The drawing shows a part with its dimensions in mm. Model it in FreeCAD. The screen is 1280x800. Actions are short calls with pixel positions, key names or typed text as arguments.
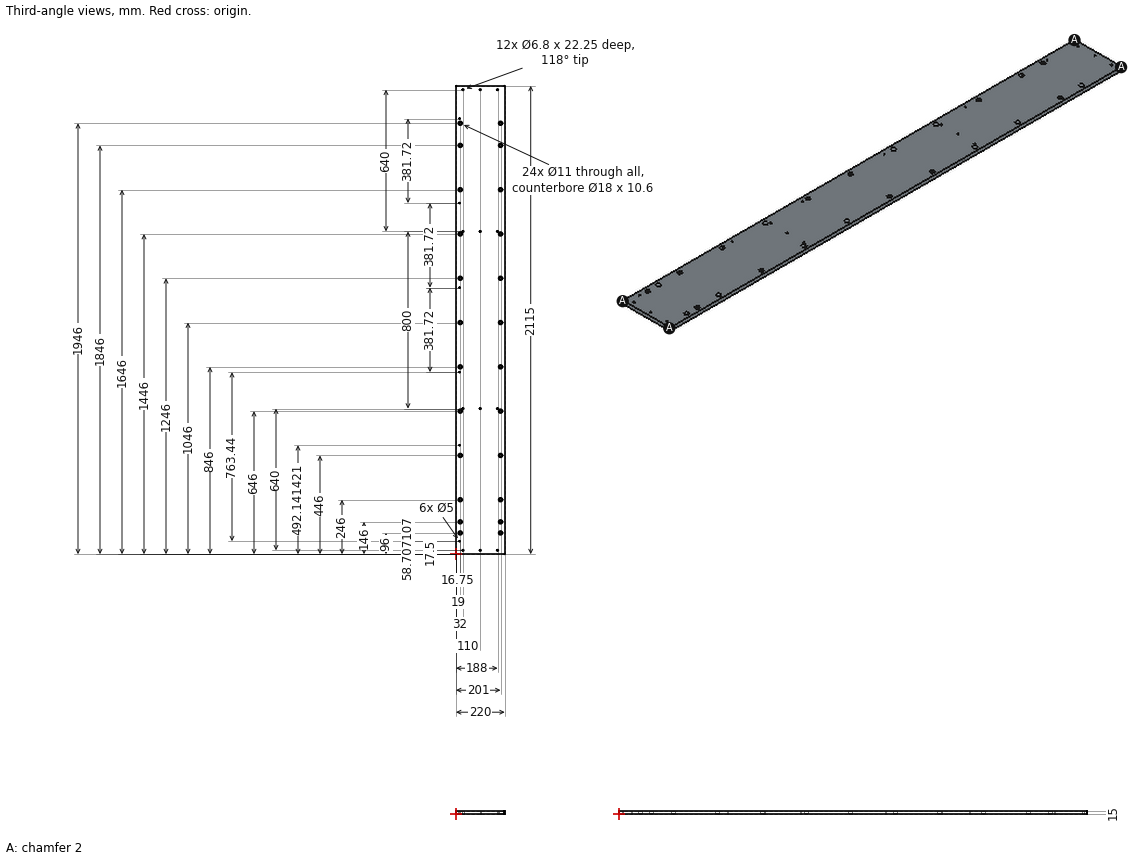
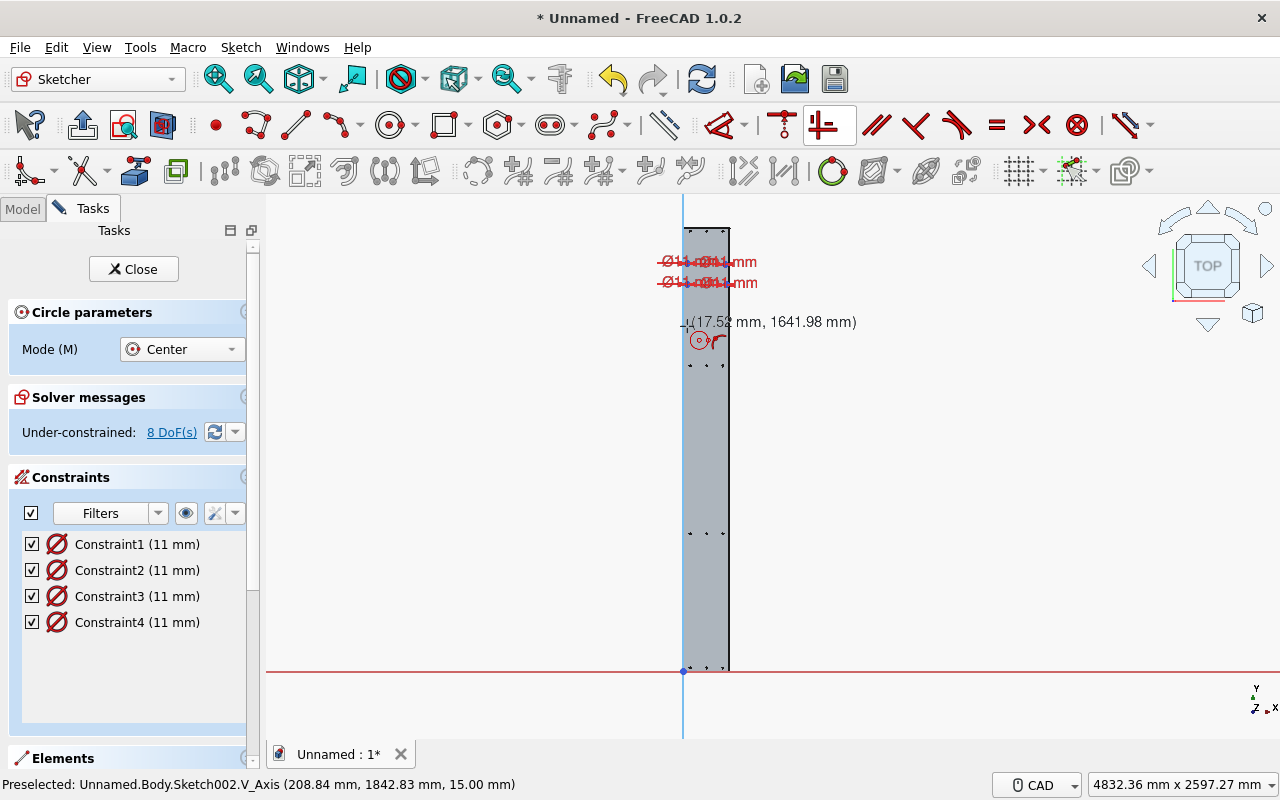
scroll(687, 326, up, 7)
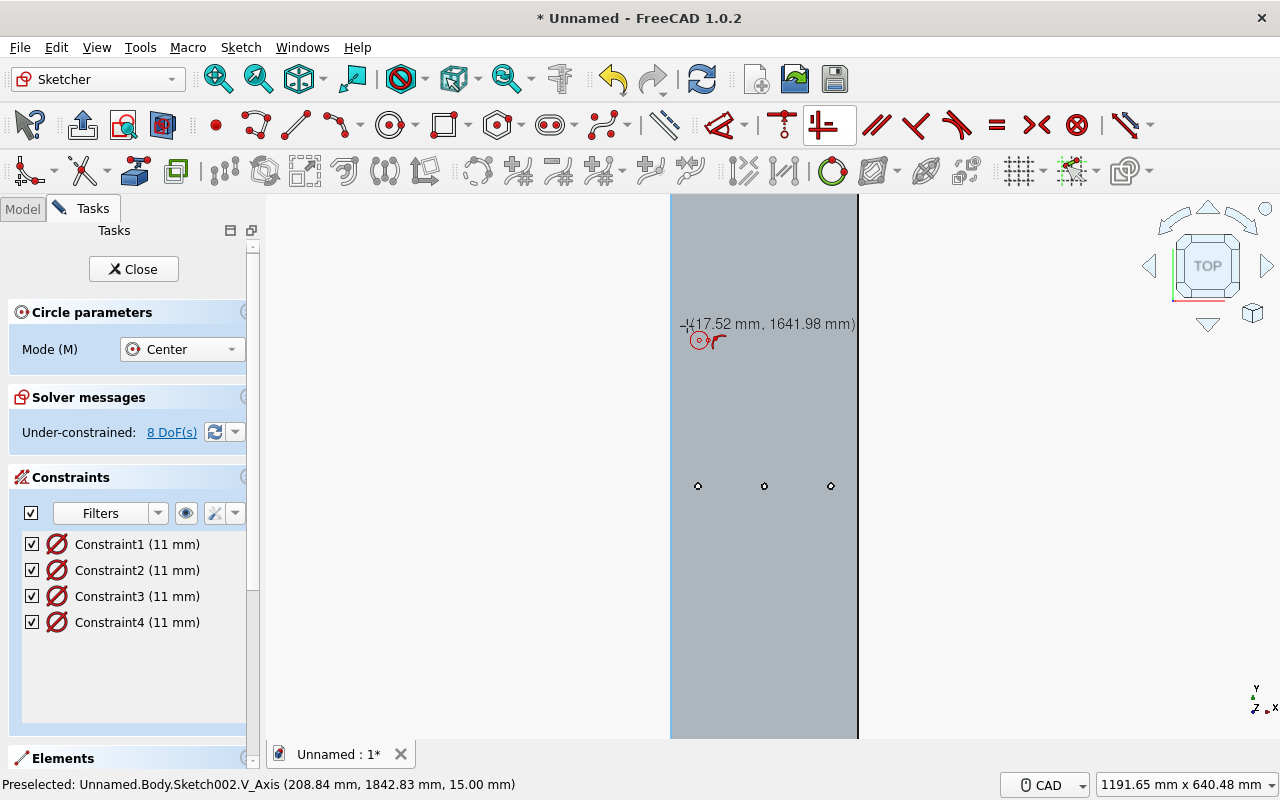
click(687, 326)
move(690, 323)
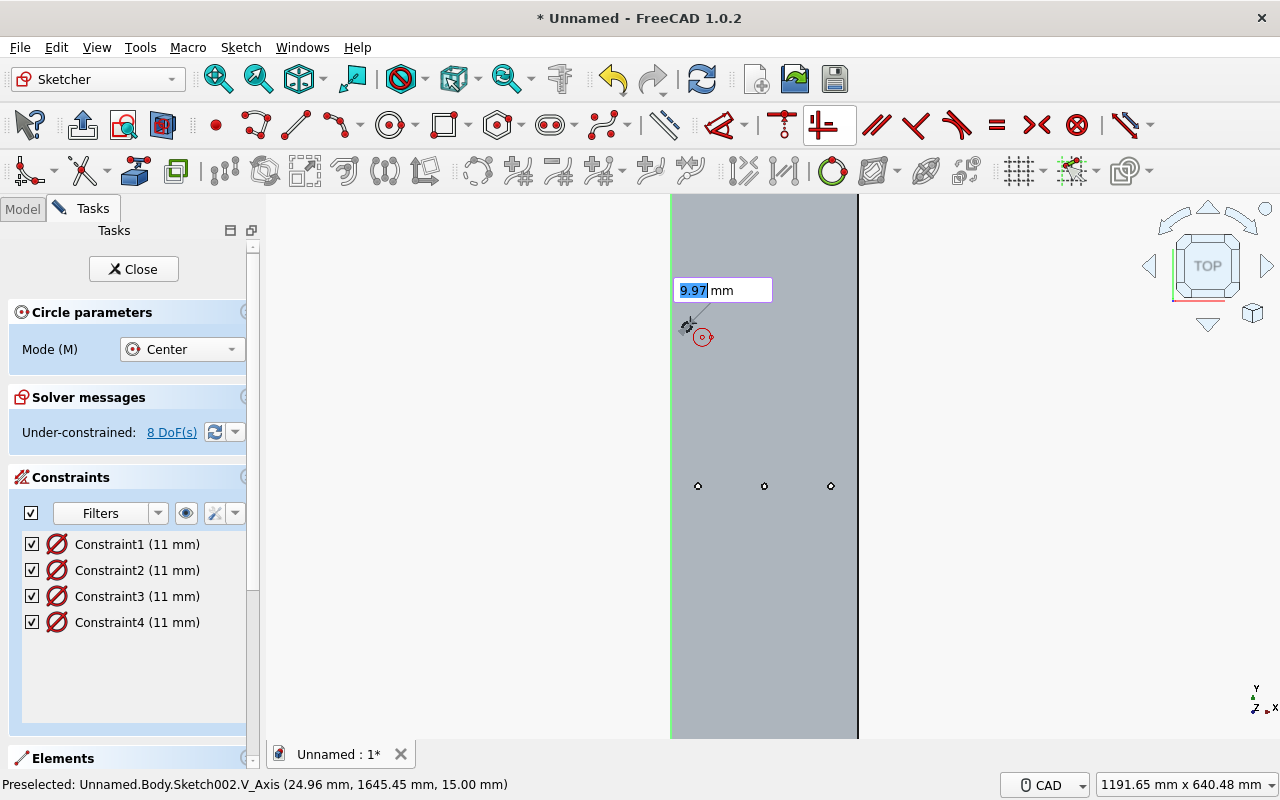
text(11)
key(Return)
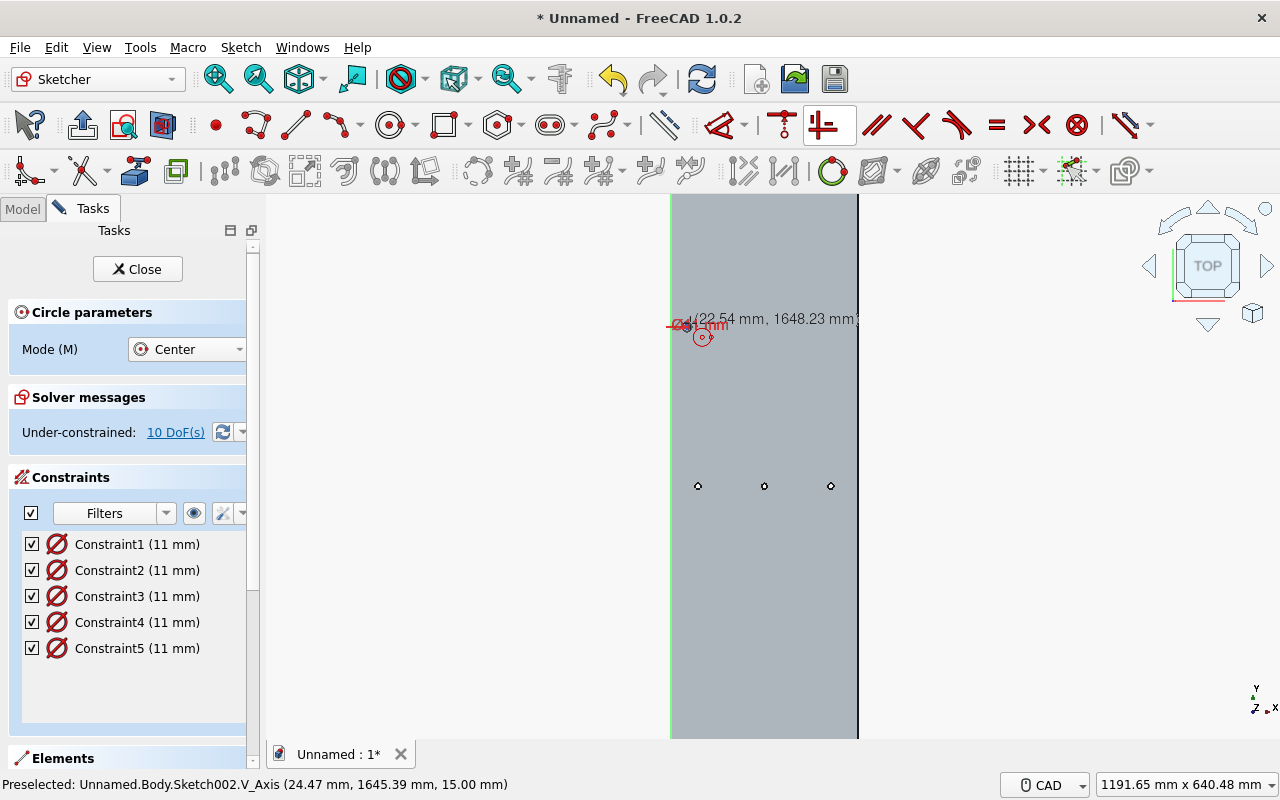
scroll(842, 326, up, 8)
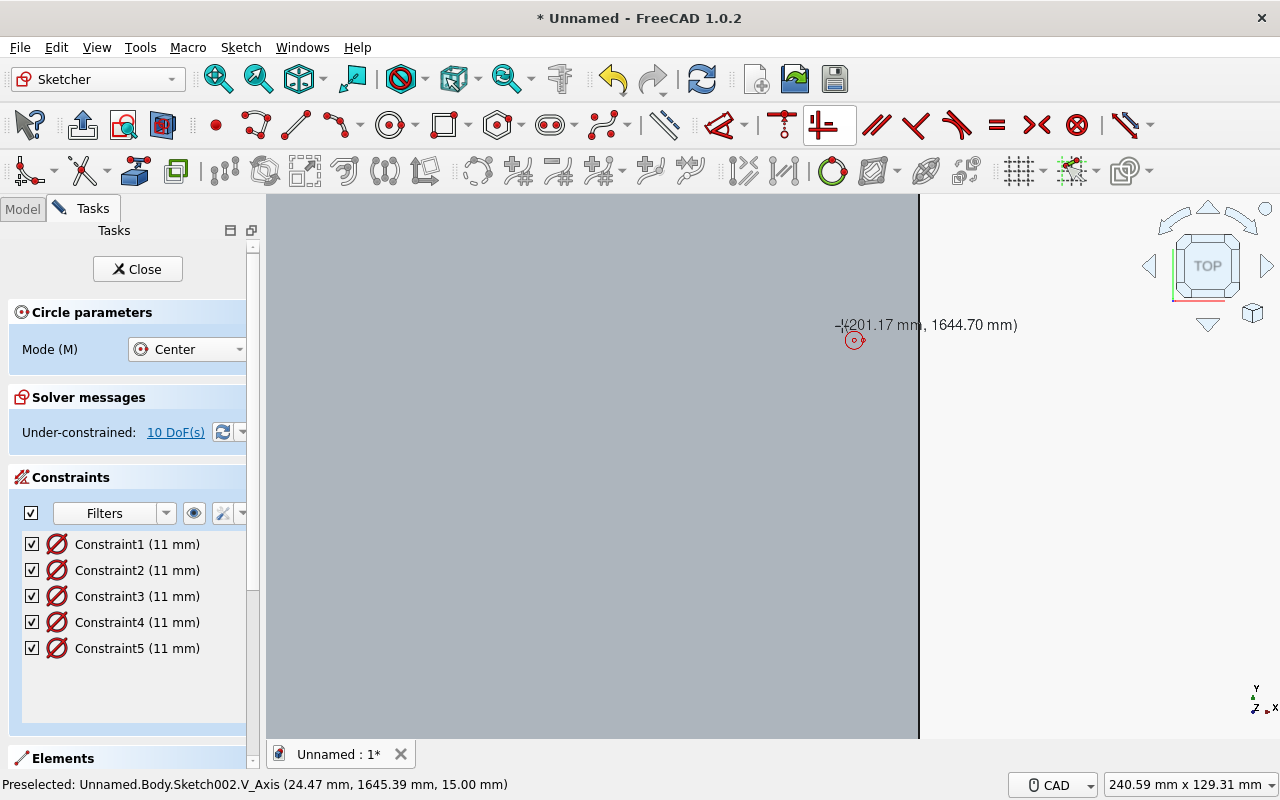
scroll(719, 326, down, 15)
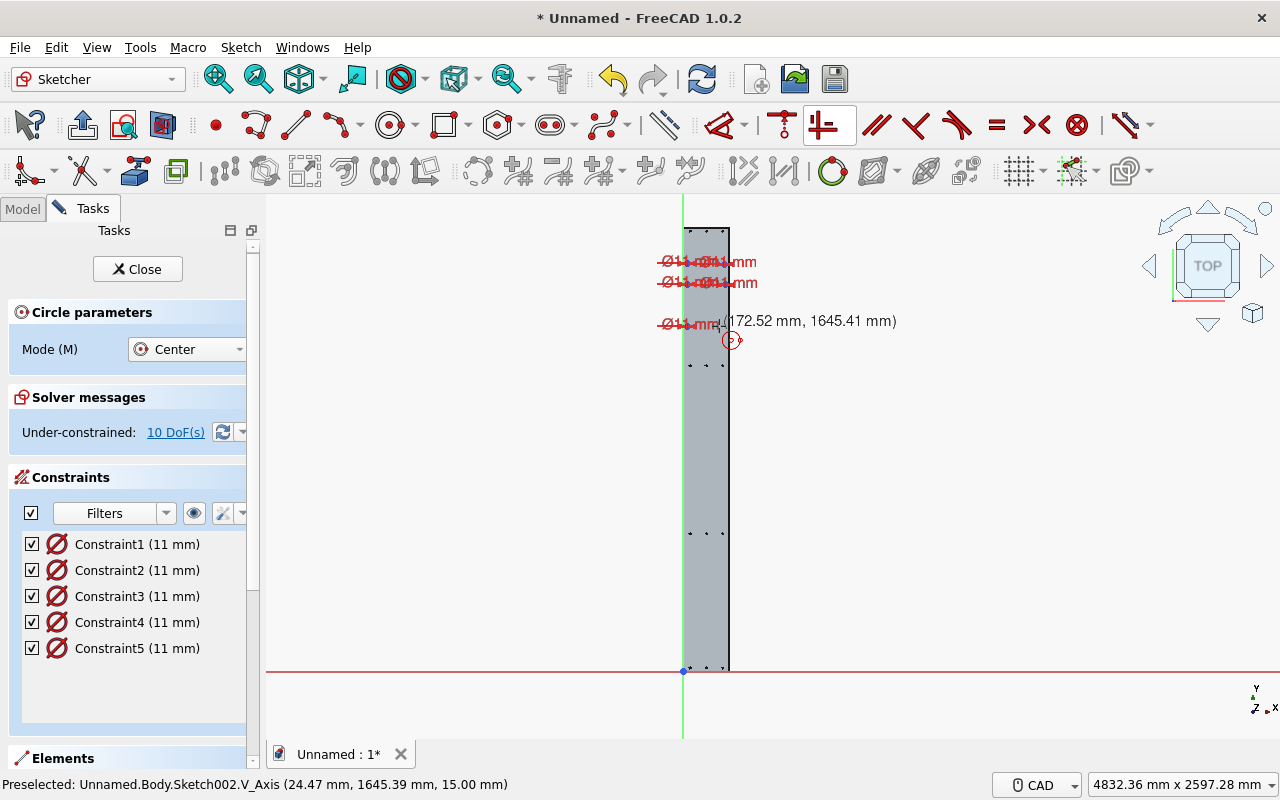
click(725, 326)
move(726, 325)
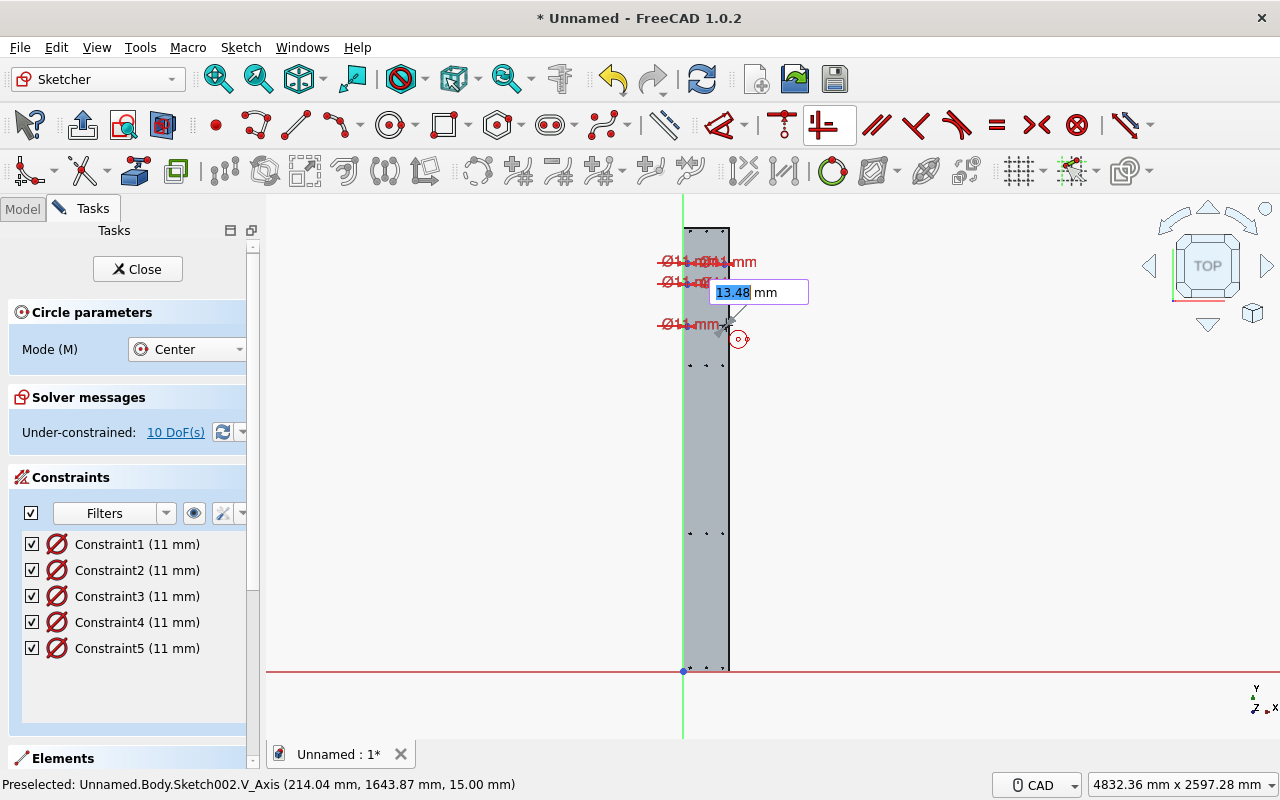
text(11)
key(Return)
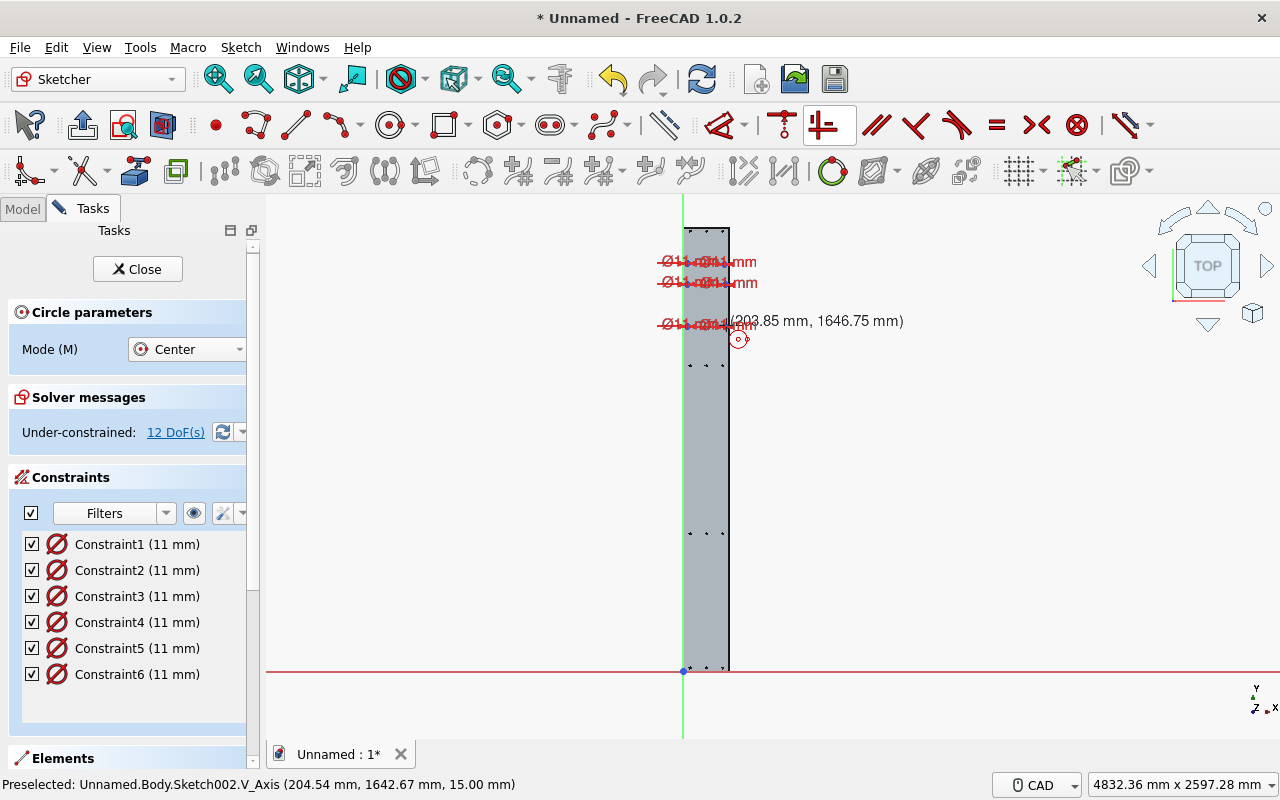
scroll(687, 368, up, 15)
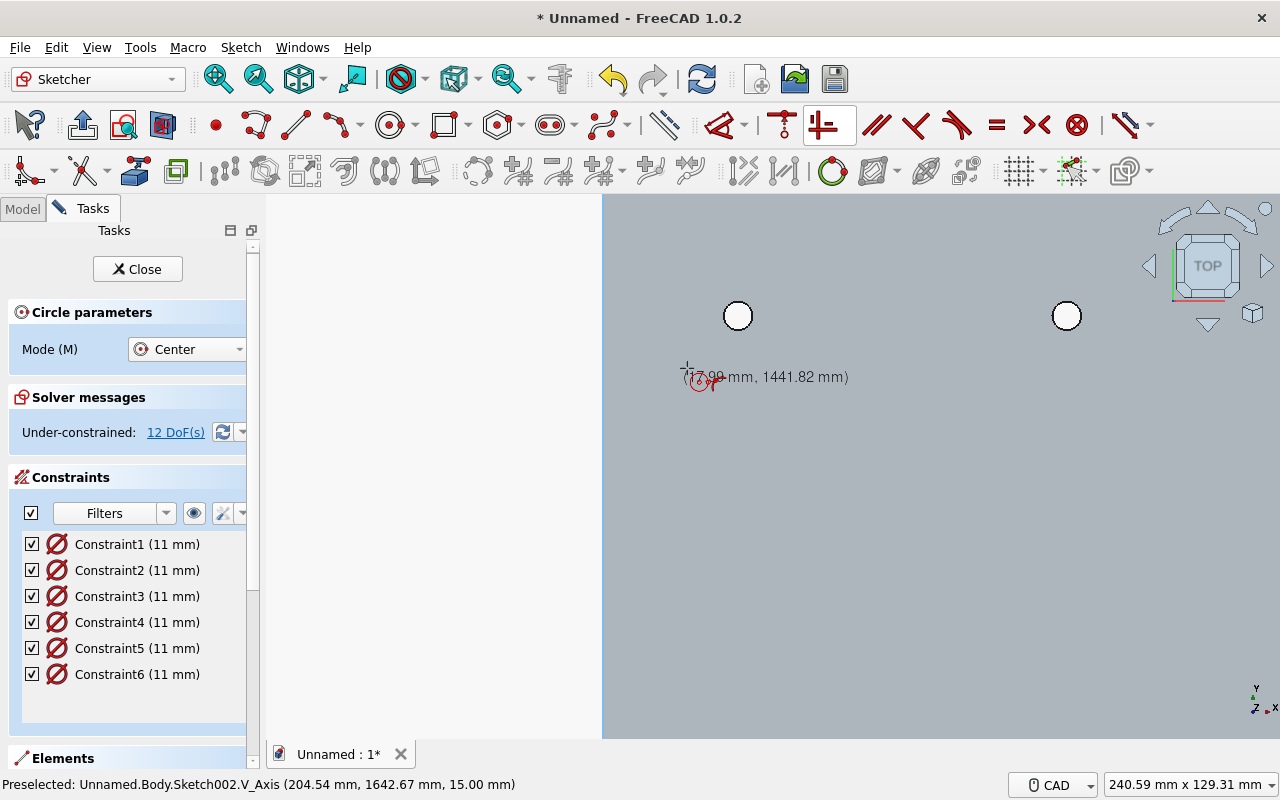
scroll(687, 368, down, 15)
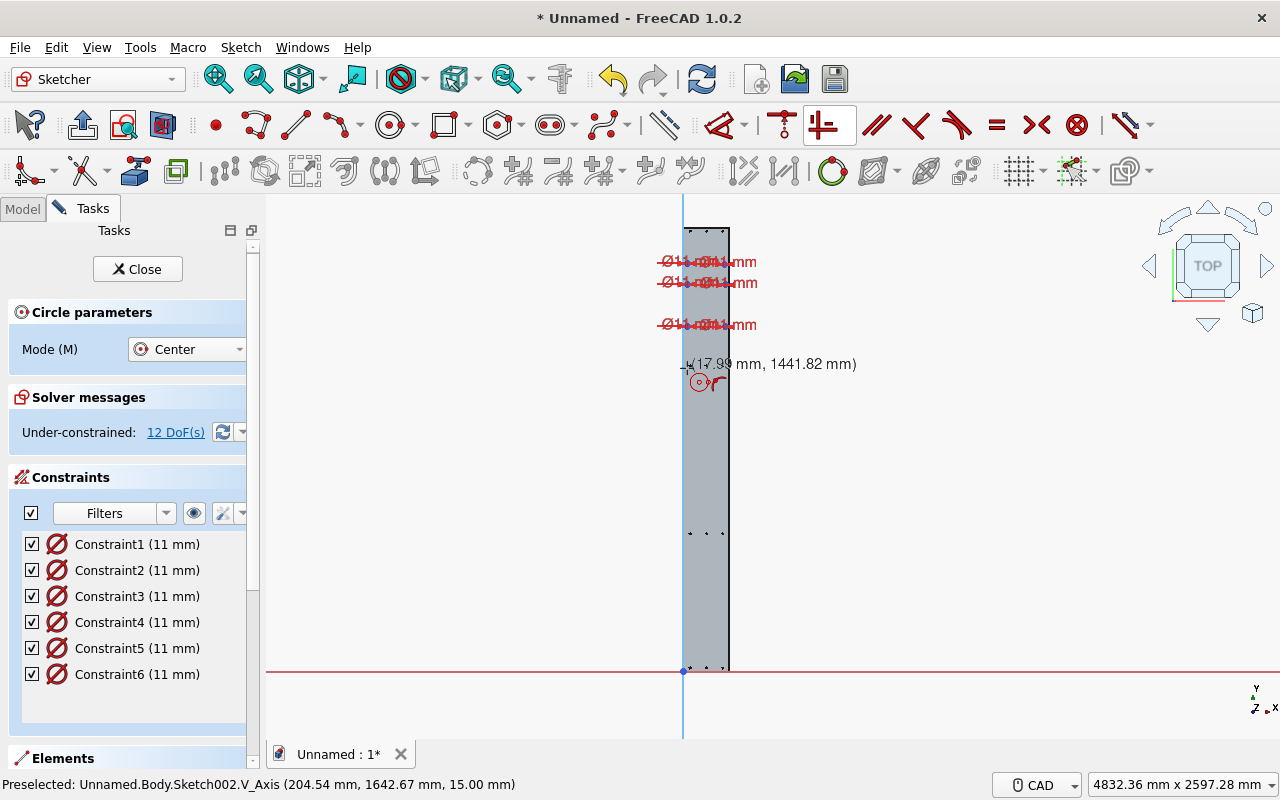
scroll(687, 368, up, 7)